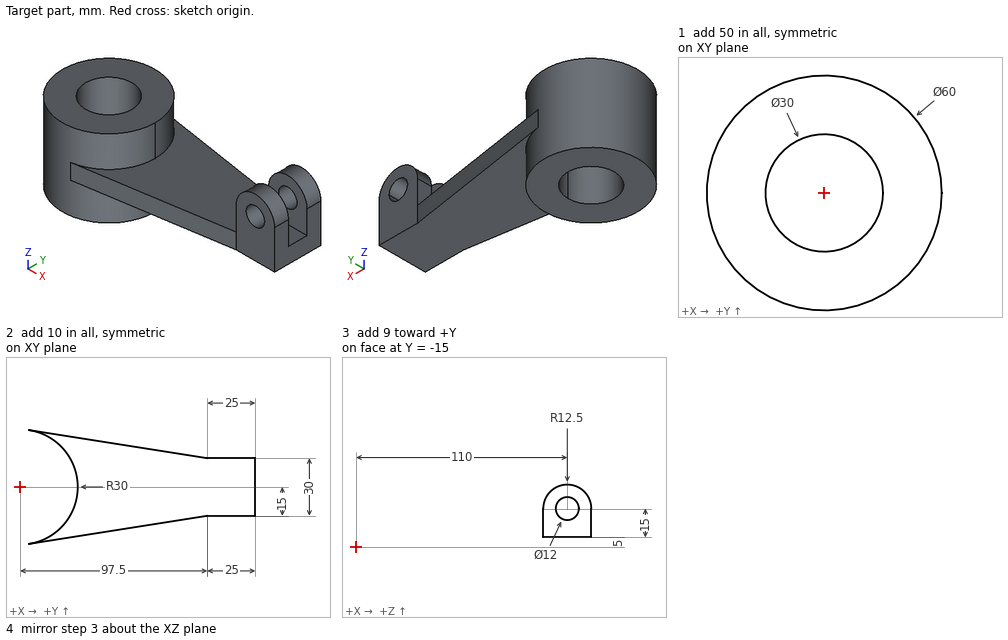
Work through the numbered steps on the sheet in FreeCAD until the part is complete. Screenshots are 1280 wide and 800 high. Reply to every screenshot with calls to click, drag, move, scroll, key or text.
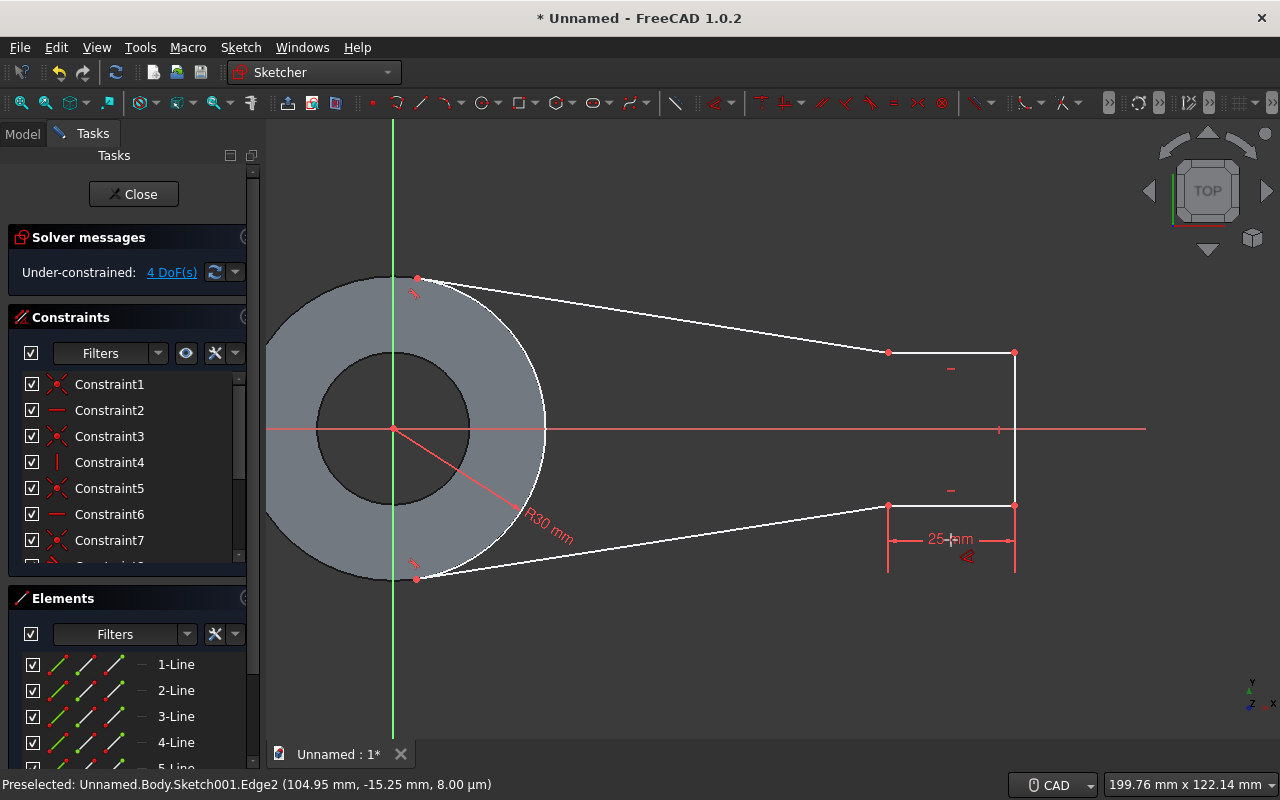
click(1015, 460)
click(1049, 394)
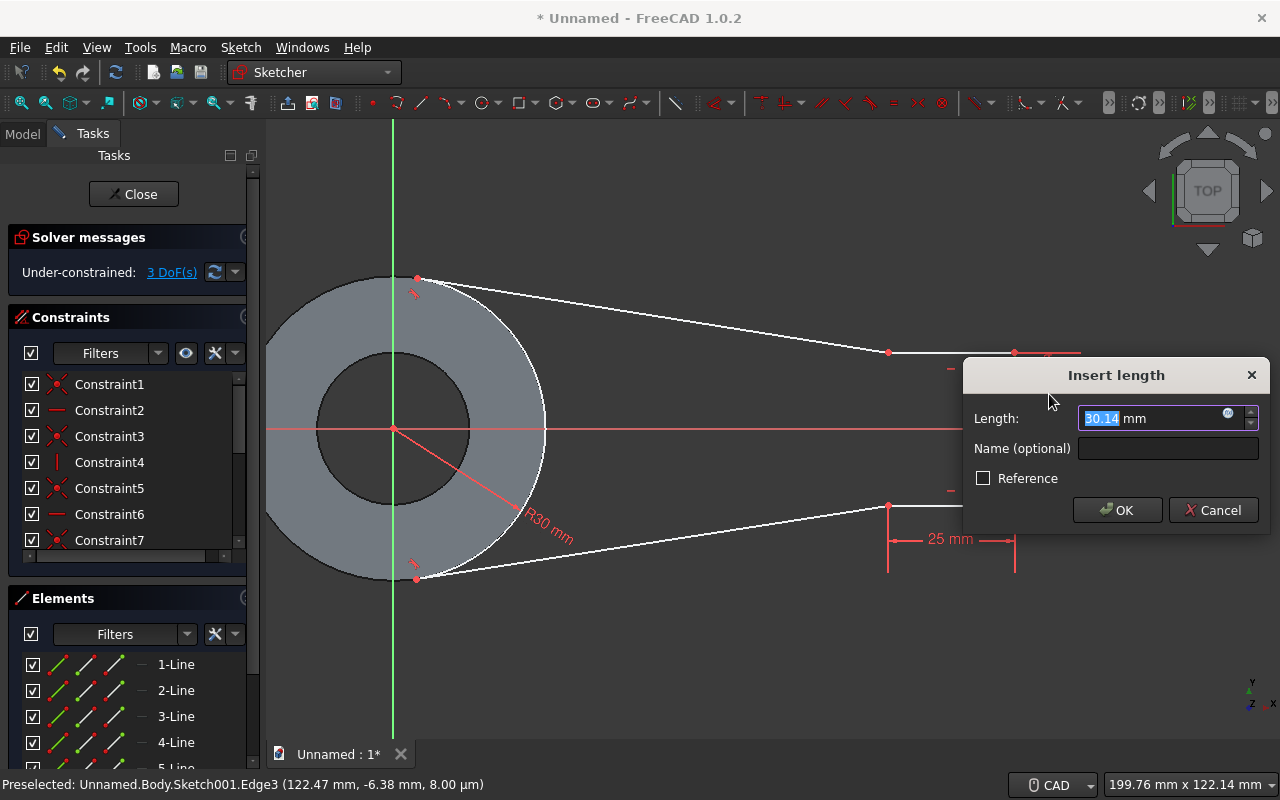
text(30)
key(Return)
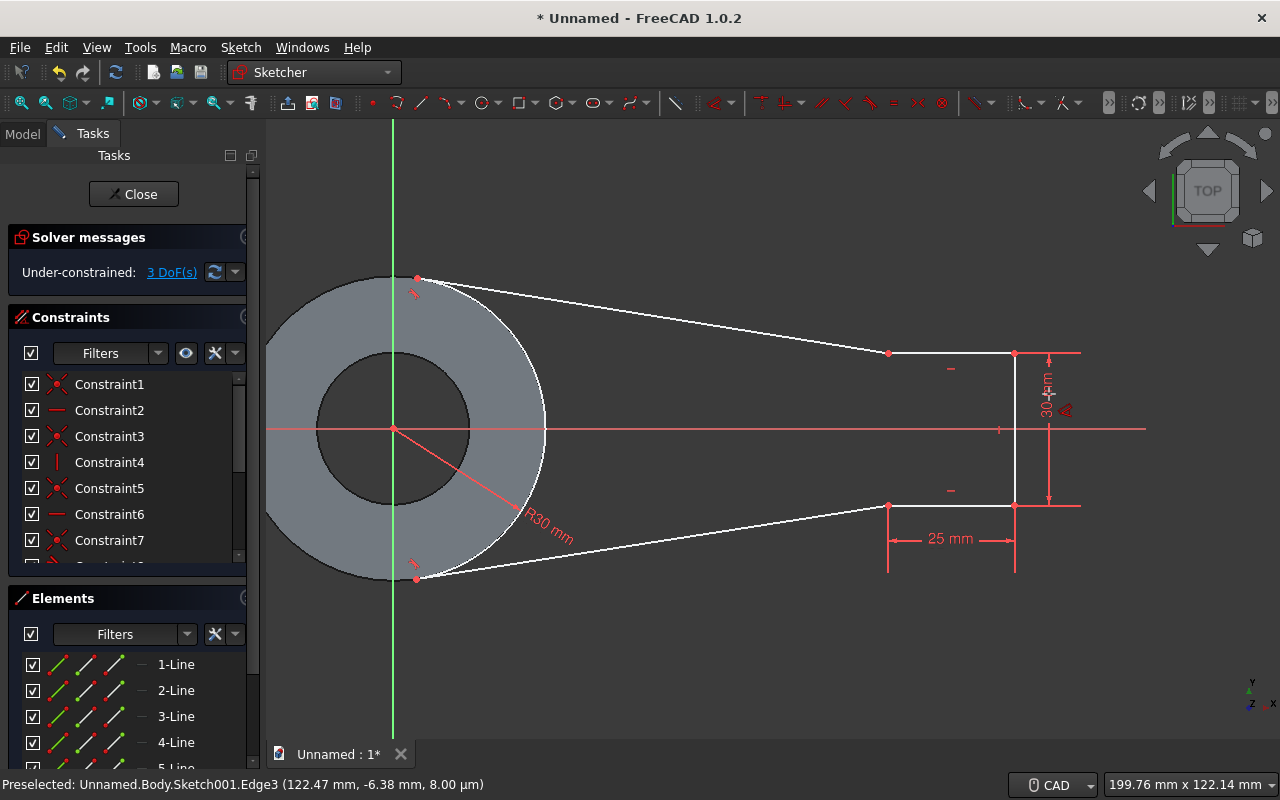
click(977, 353)
click(951, 319)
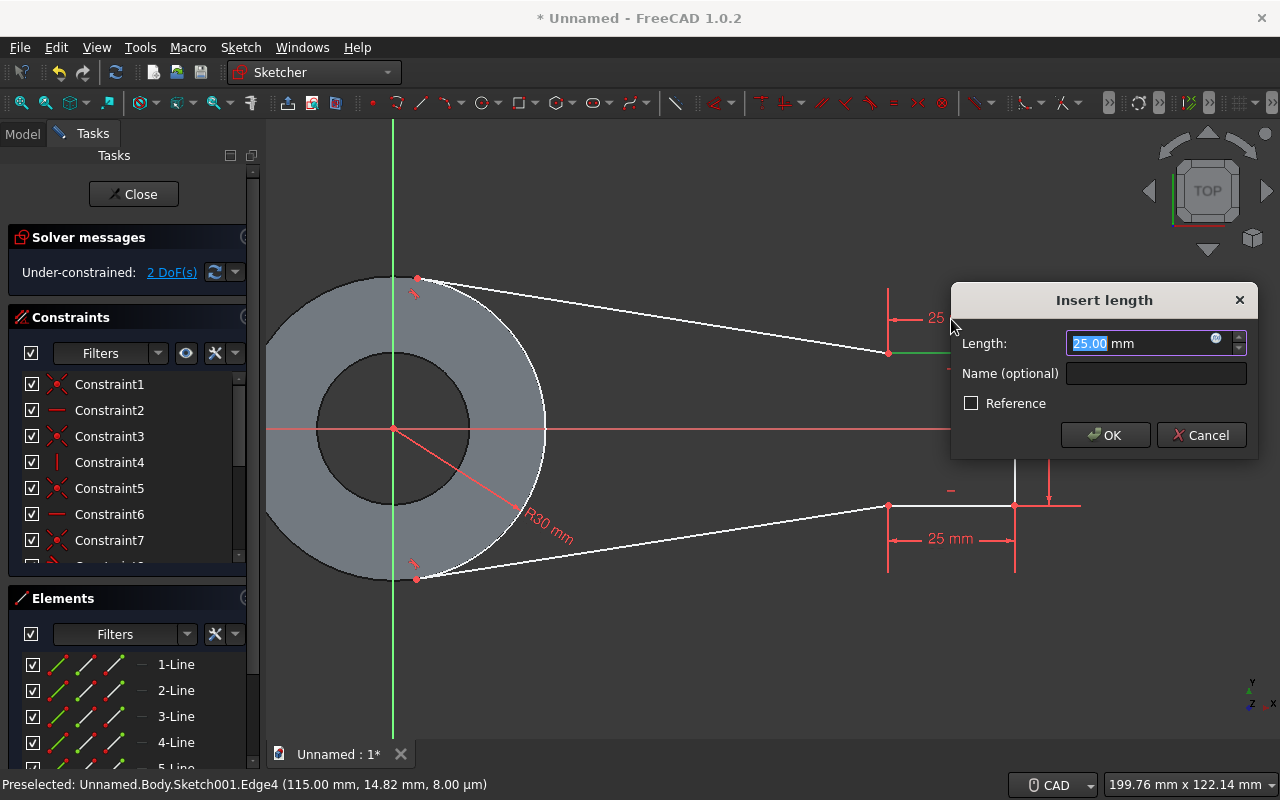
text(25)
key(Return)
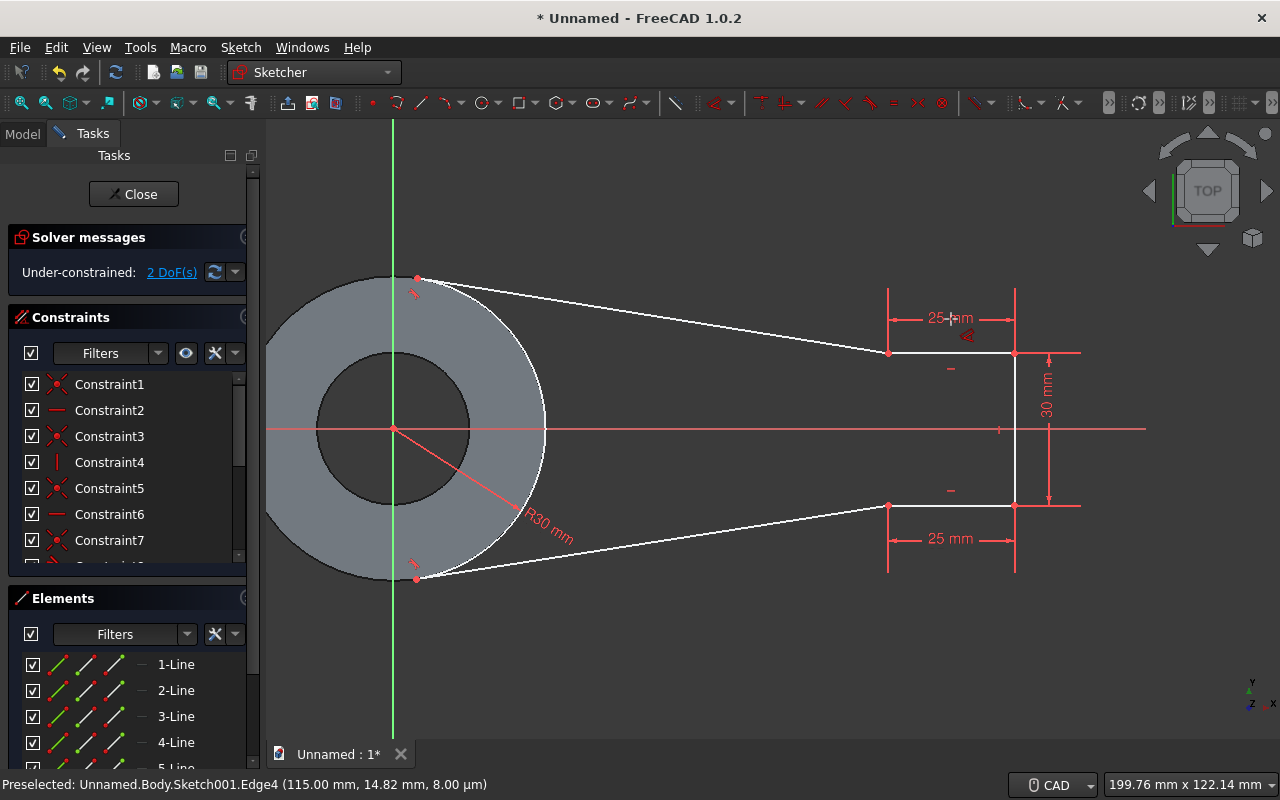
click(888, 506)
click(359, 467)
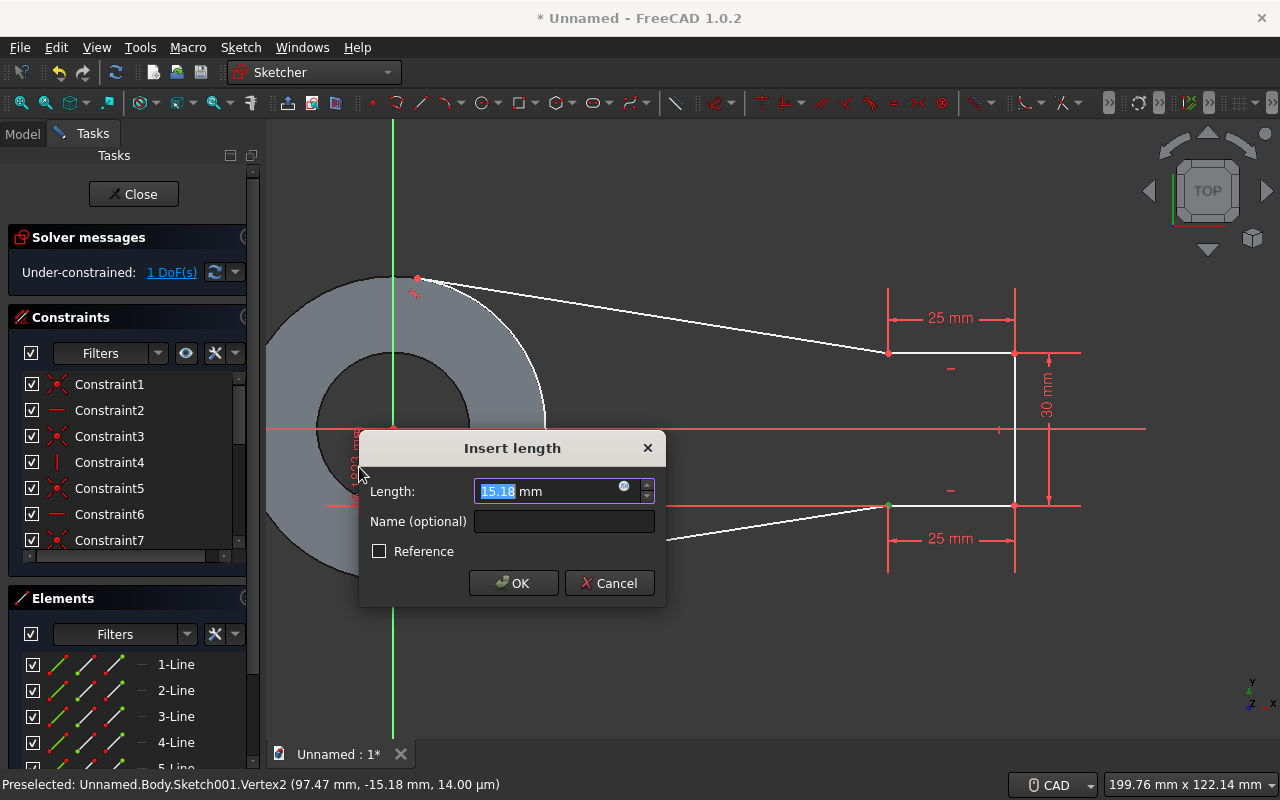
text(15)
key(Return)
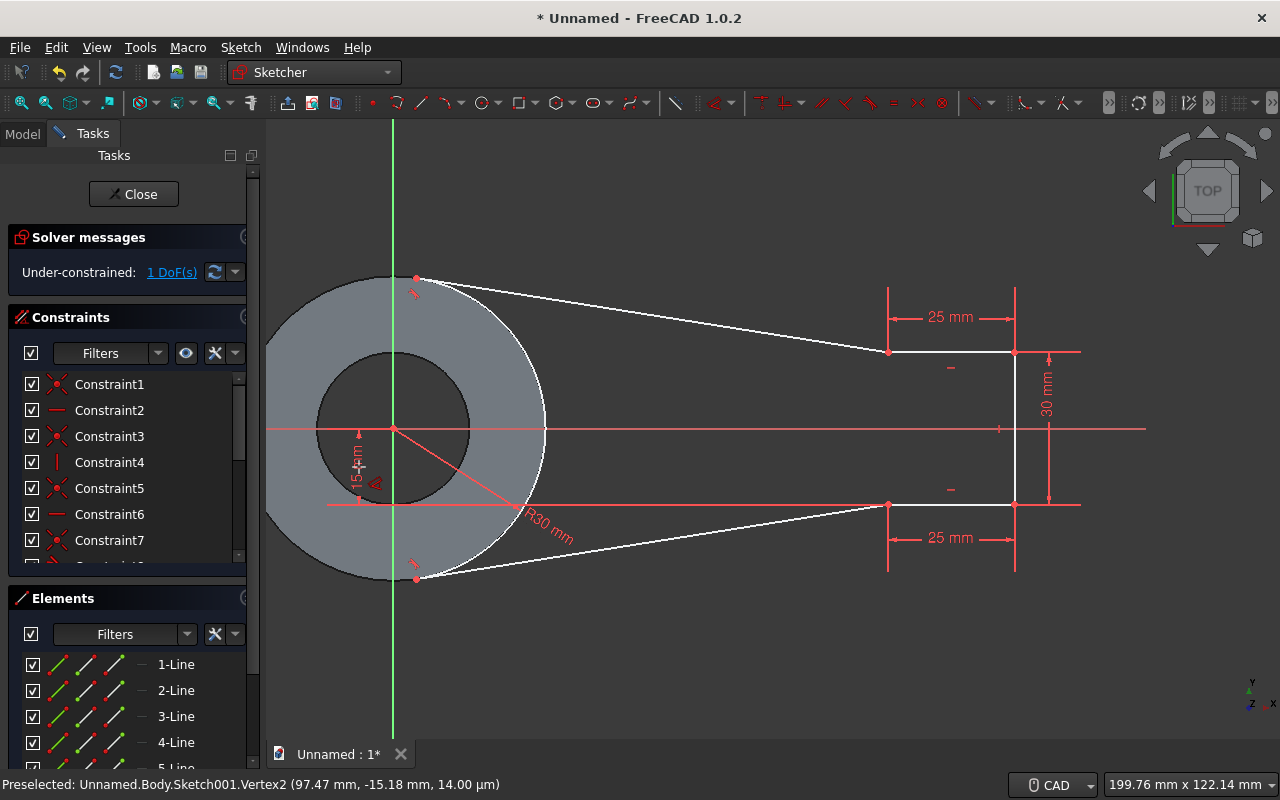
click(888, 505)
click(467, 539)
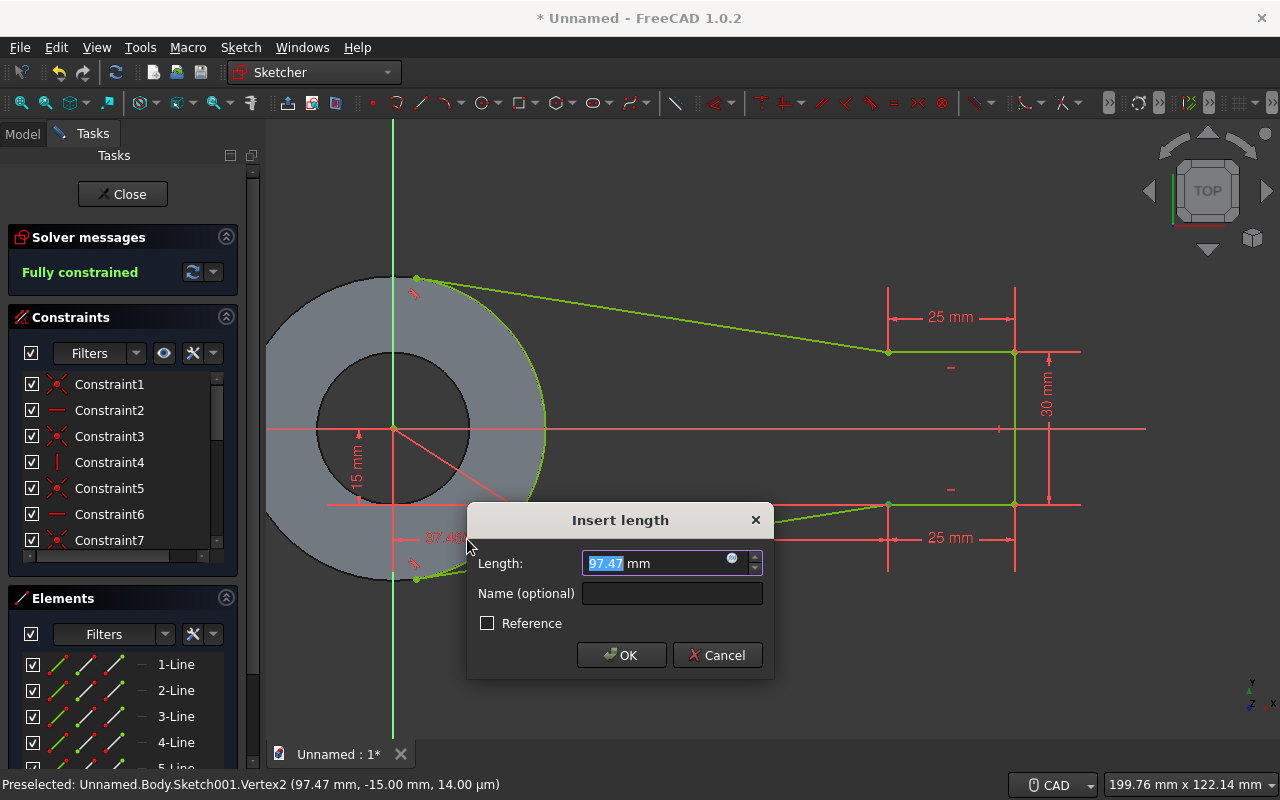
text(97.5)
key(Return)
key(Escape)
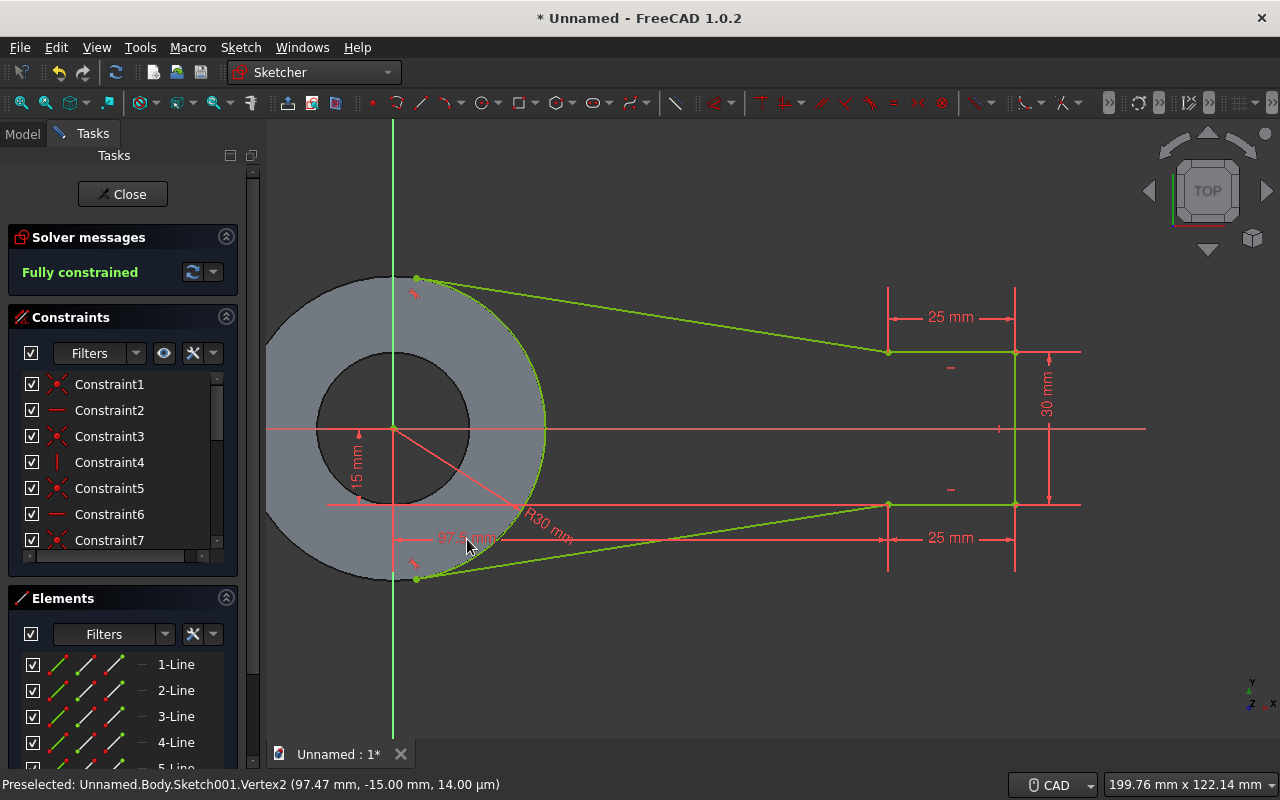
click(123, 194)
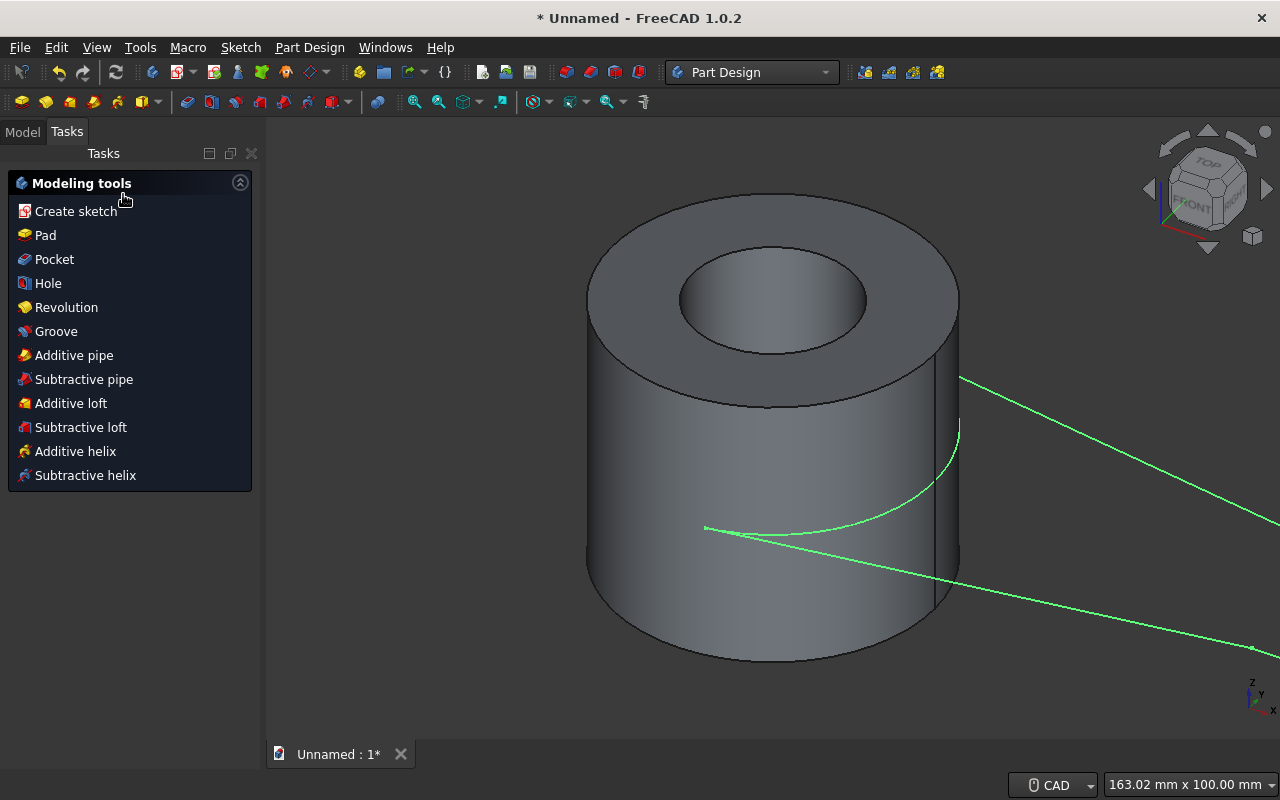
click(22, 102)